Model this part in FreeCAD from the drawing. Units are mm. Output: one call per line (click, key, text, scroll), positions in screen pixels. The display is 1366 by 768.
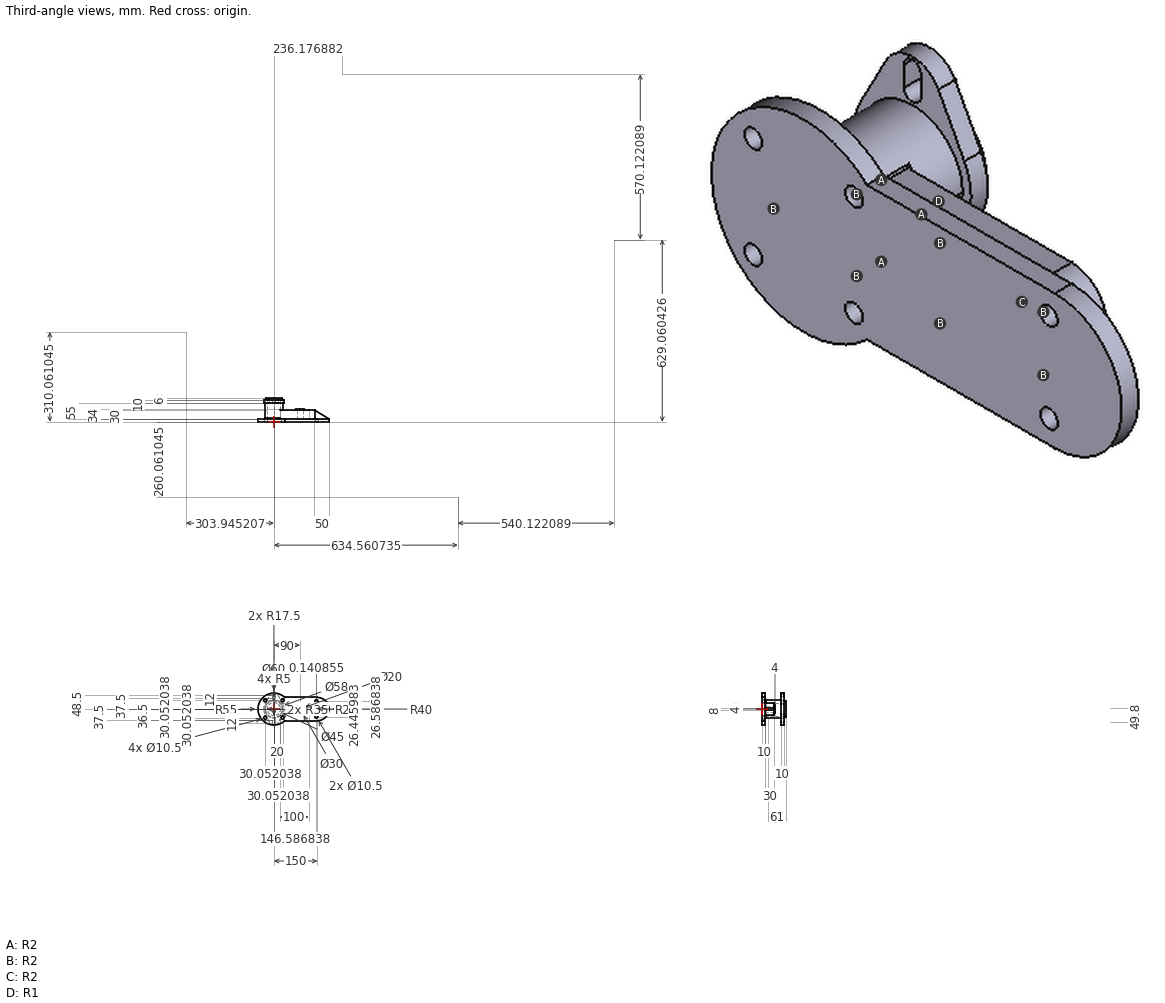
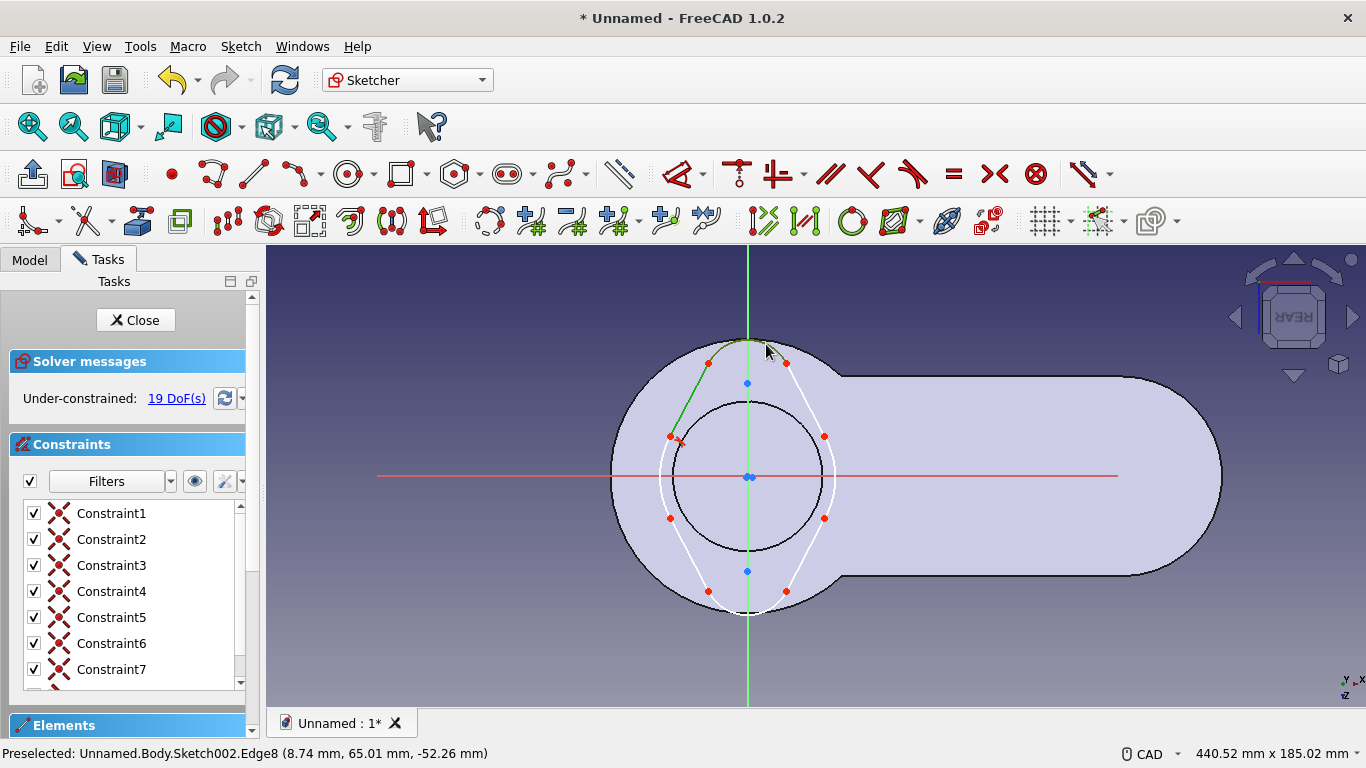
key(t)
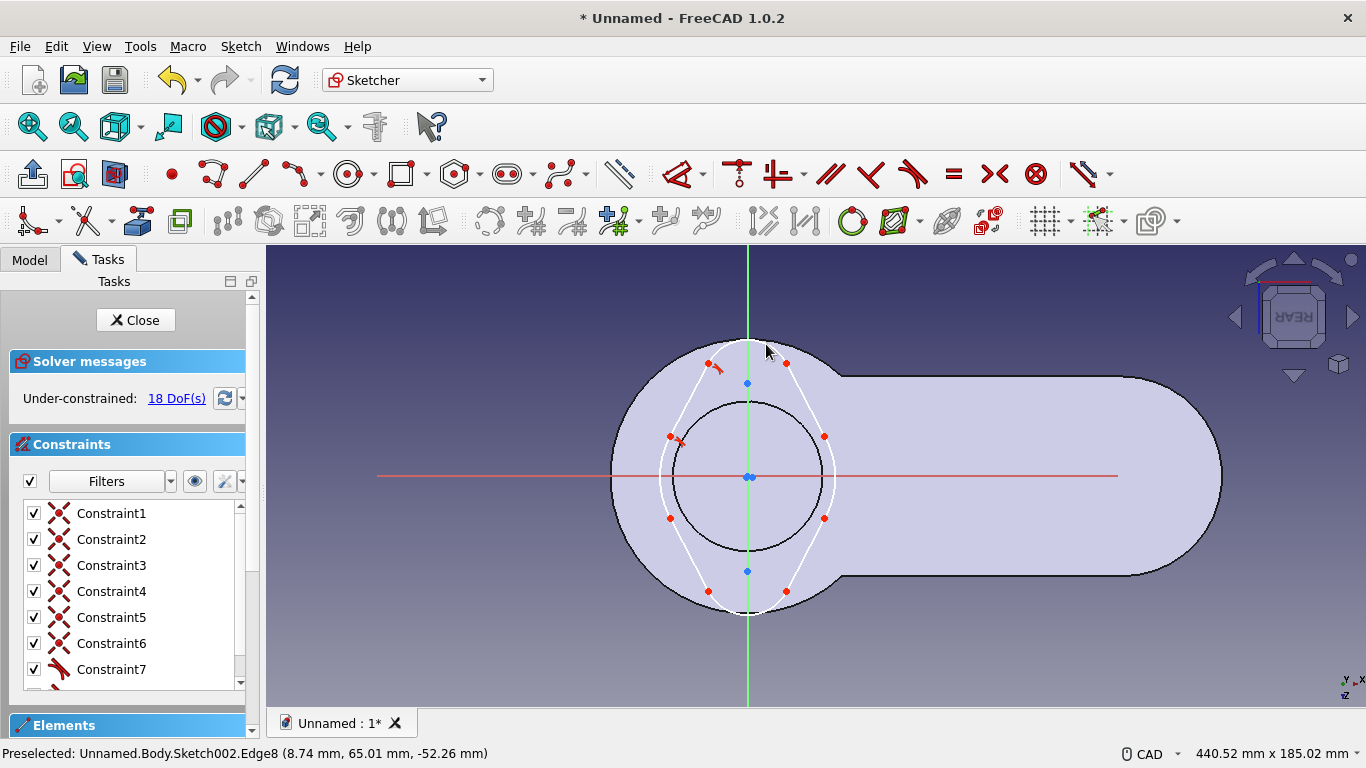
click(682, 540)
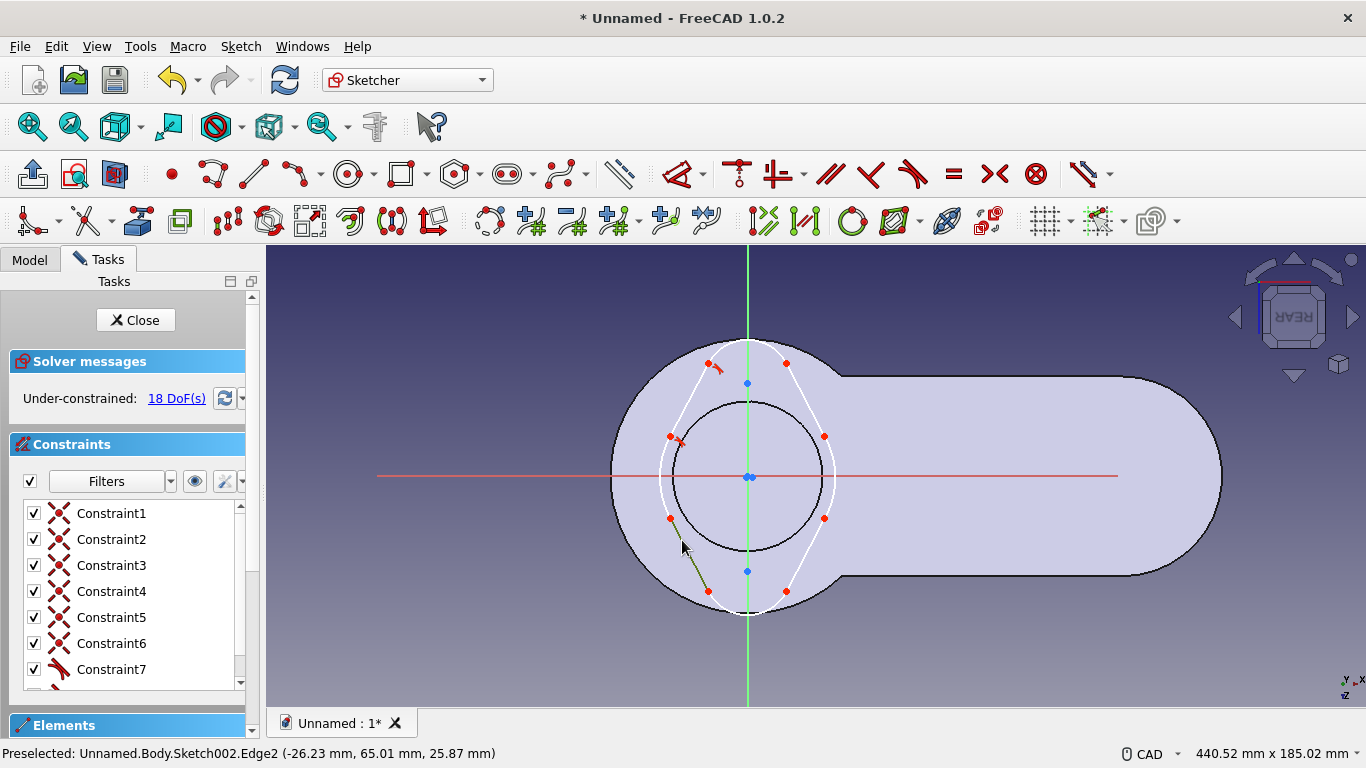
click(662, 461)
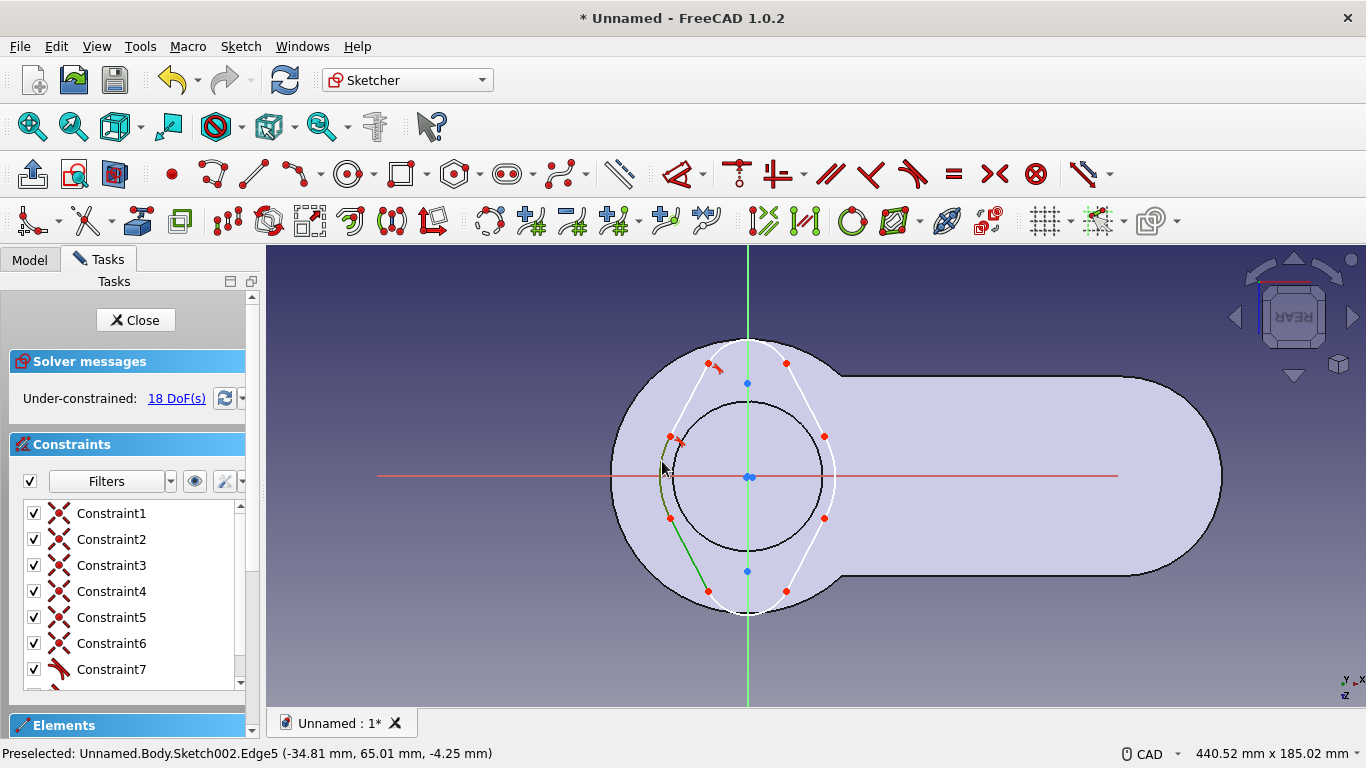
key(t)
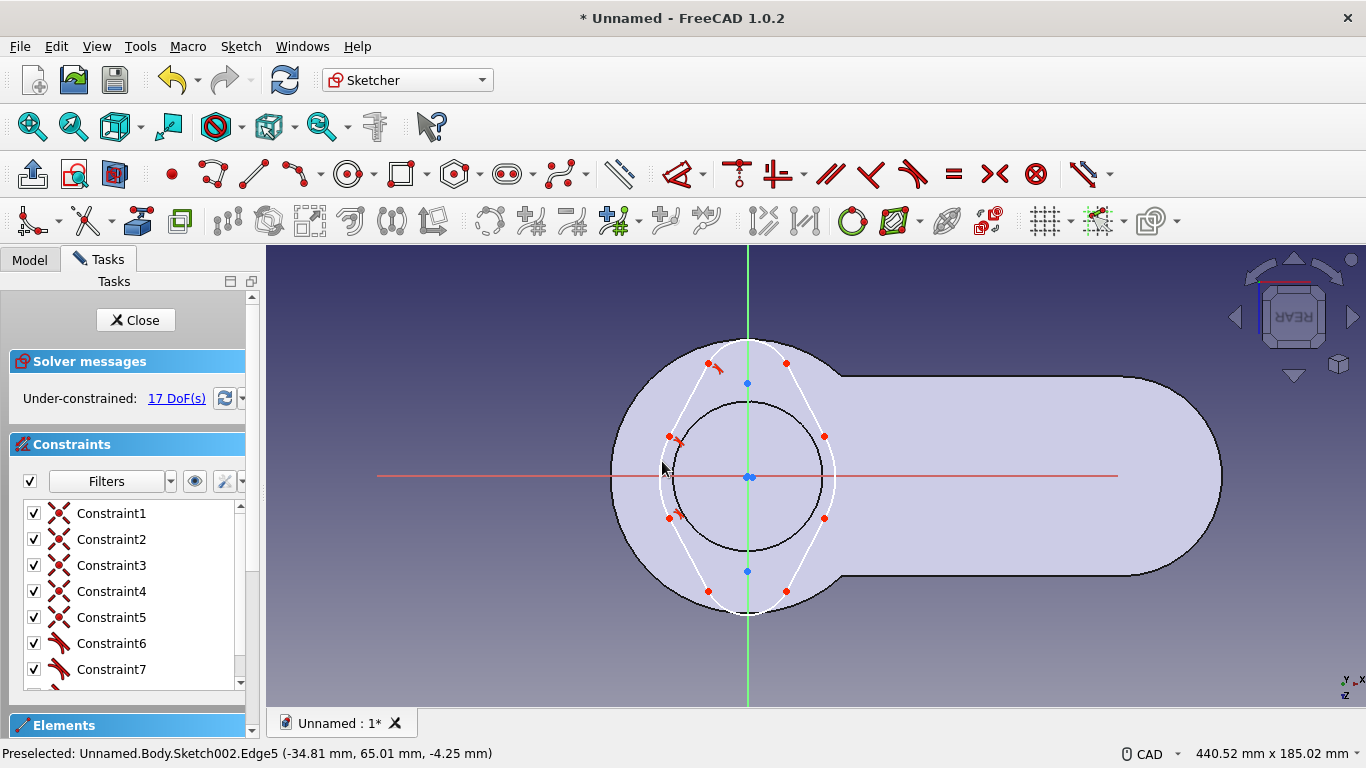
click(681, 540)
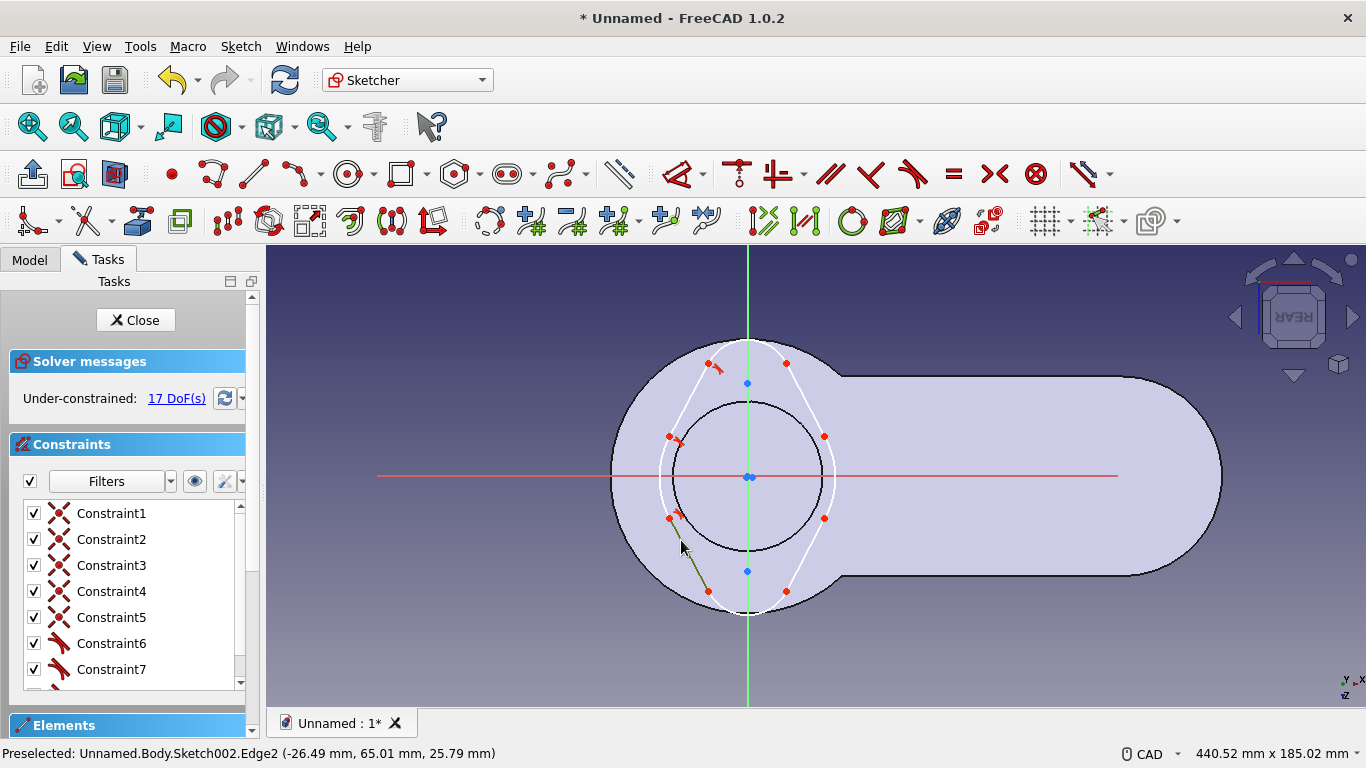
click(729, 611)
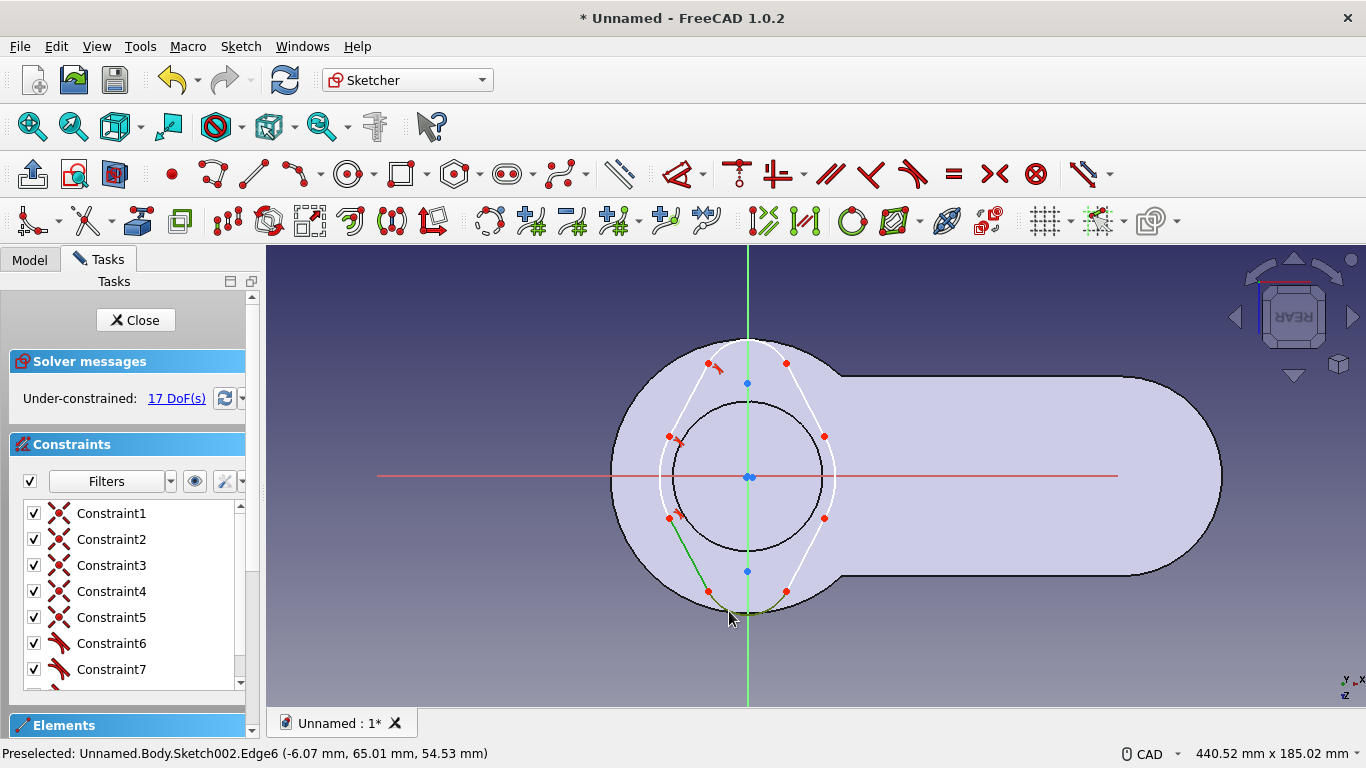
key(t)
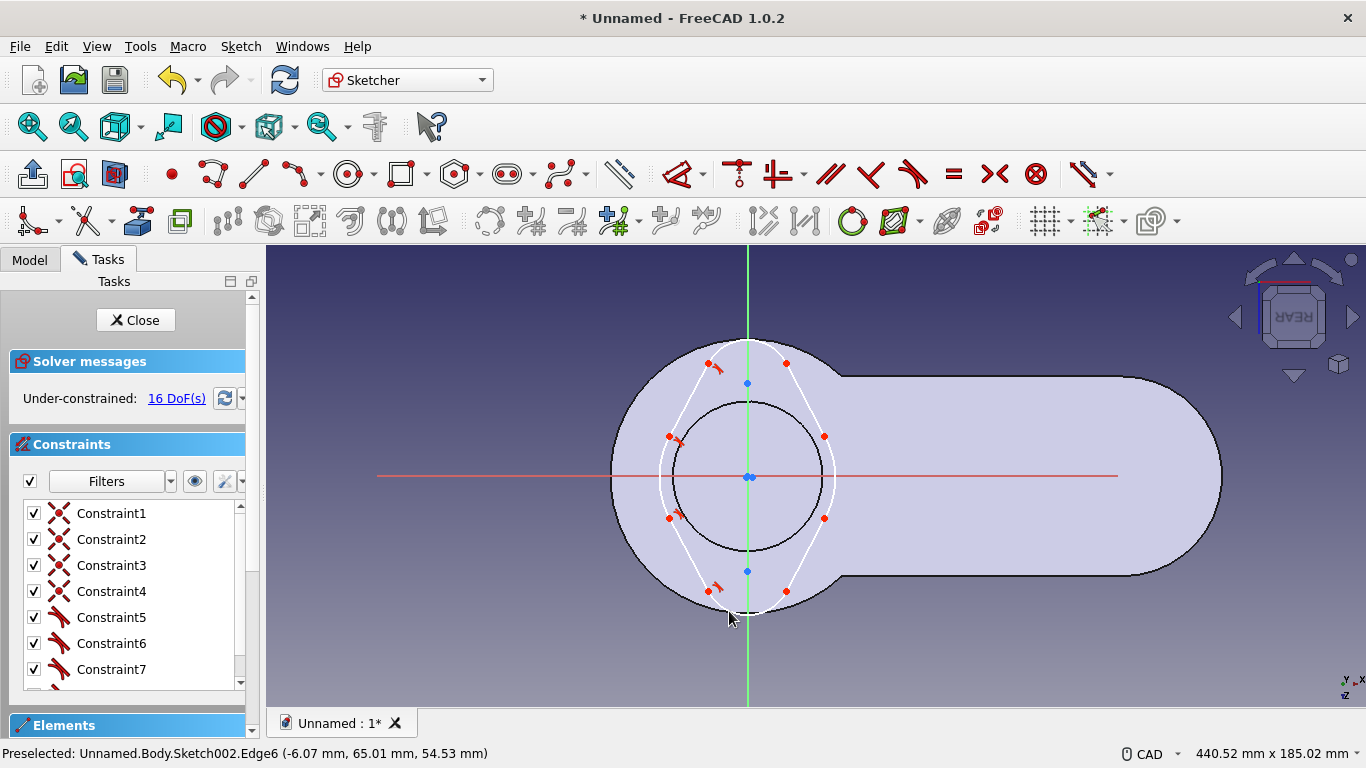
click(798, 570)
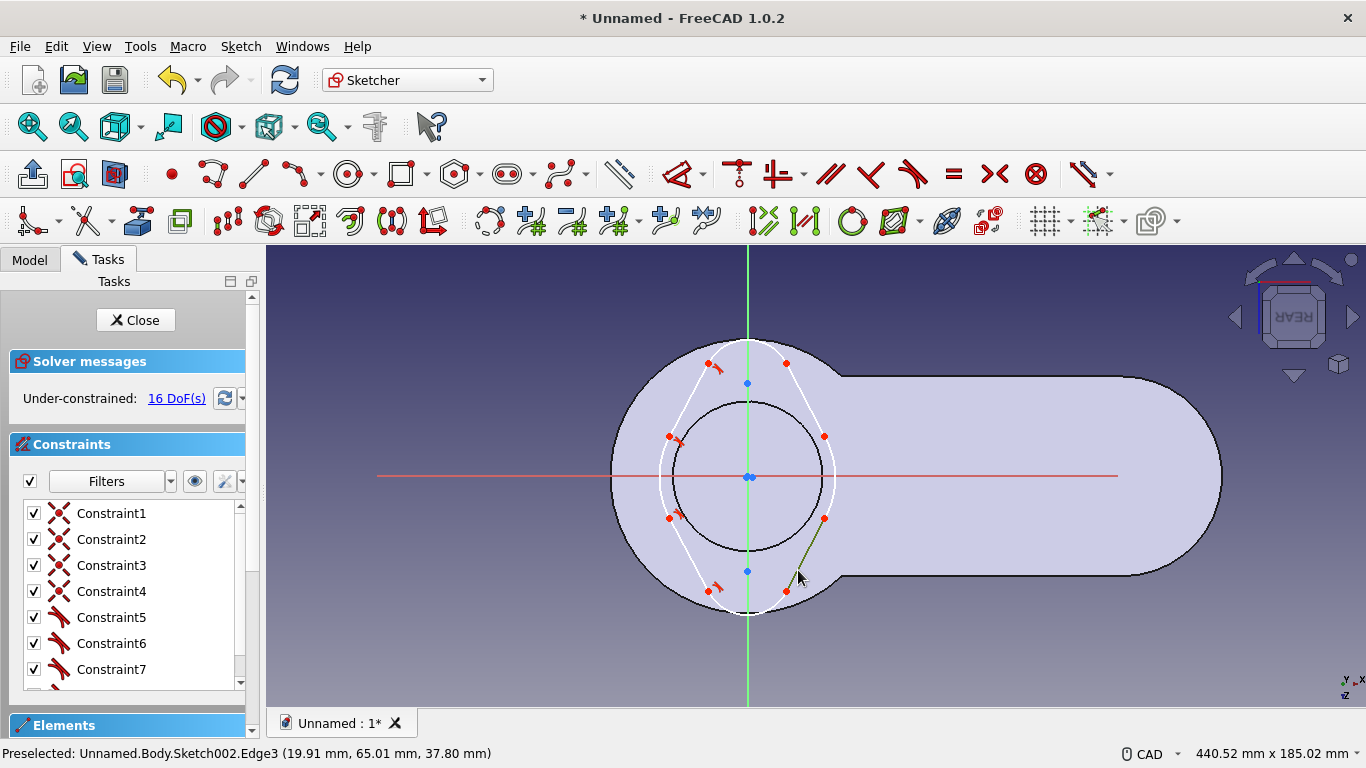
click(729, 611)